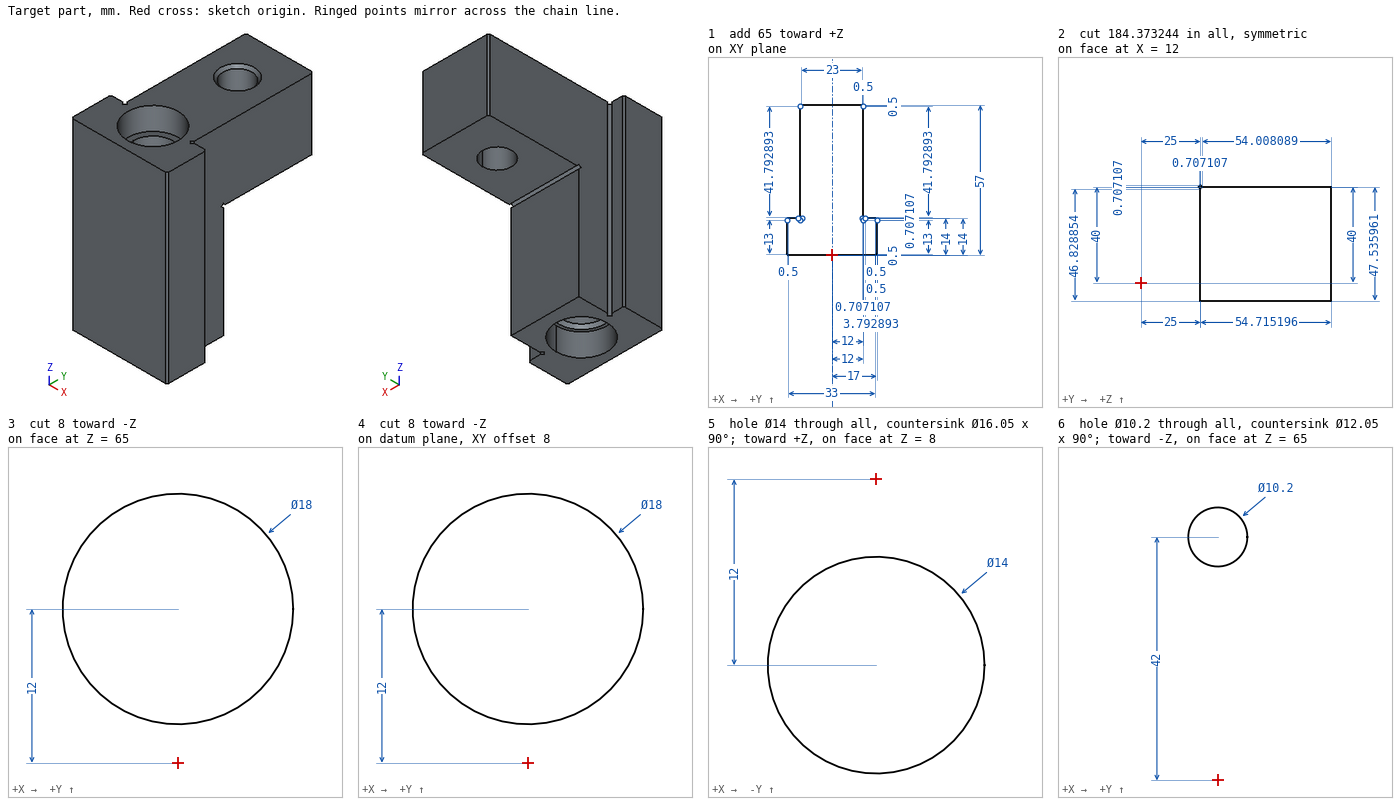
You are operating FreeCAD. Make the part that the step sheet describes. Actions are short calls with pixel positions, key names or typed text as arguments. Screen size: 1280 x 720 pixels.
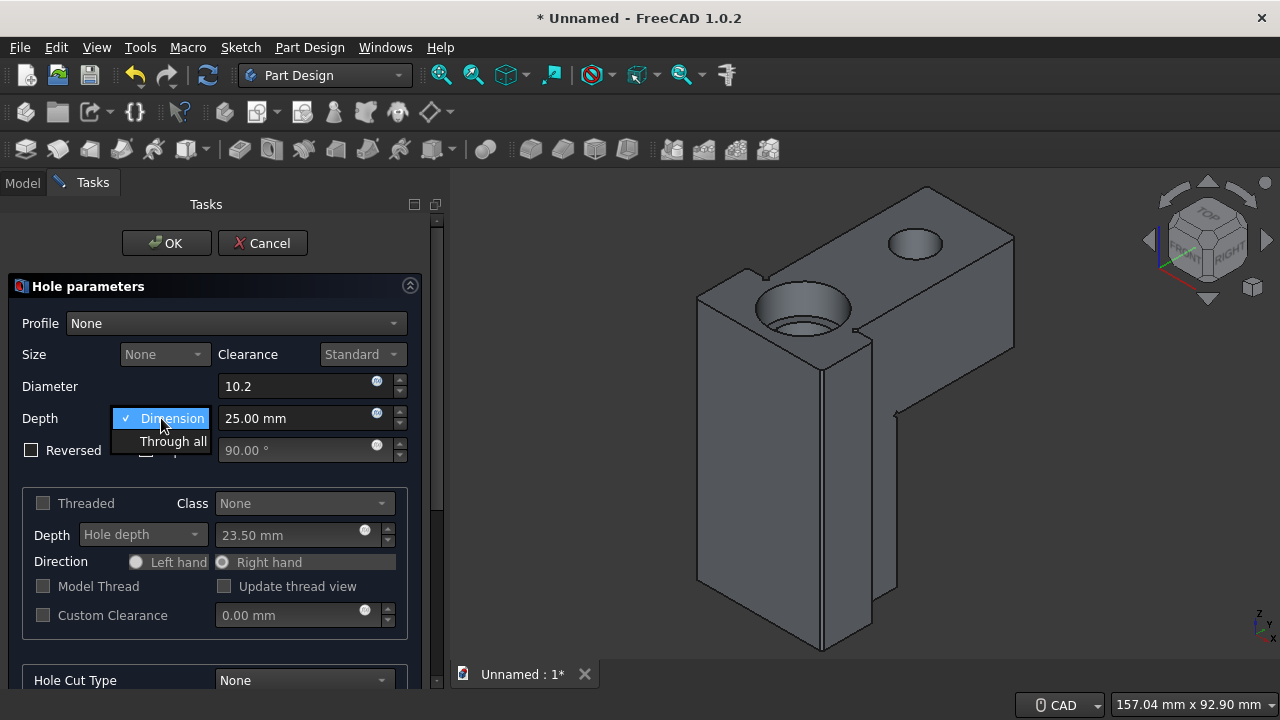
click(160, 442)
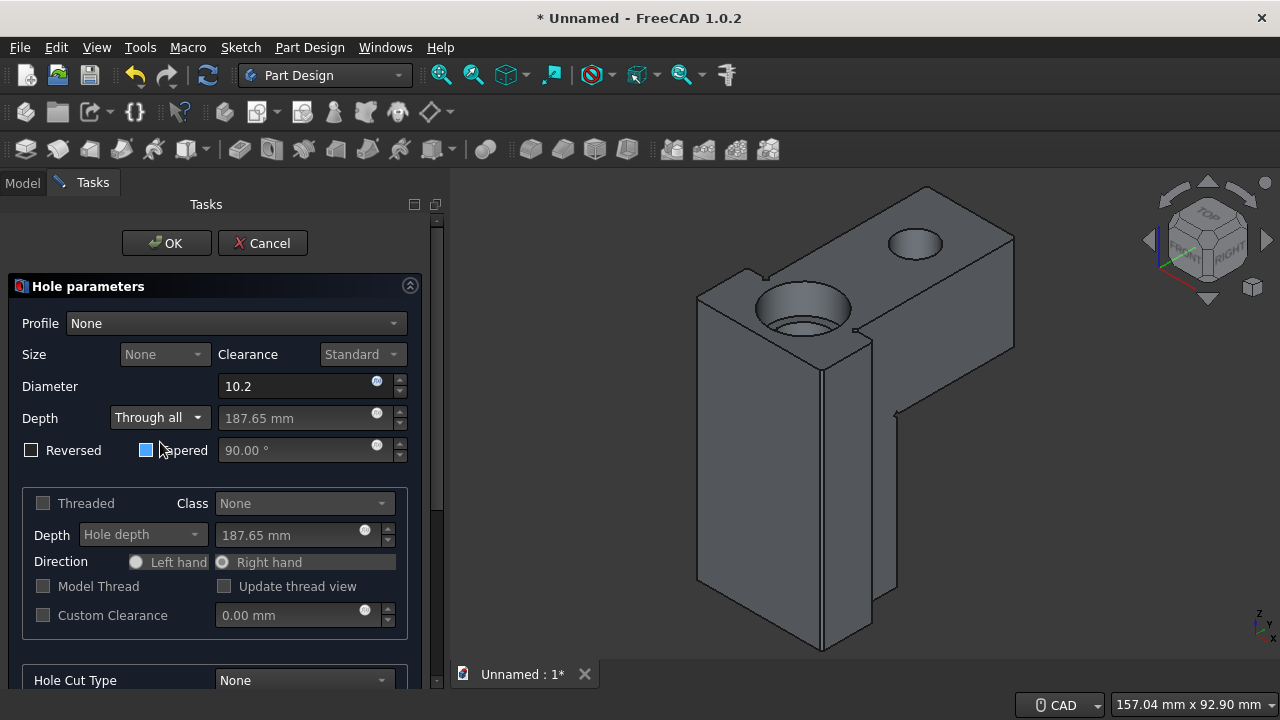
scroll(437, 451, down, 2)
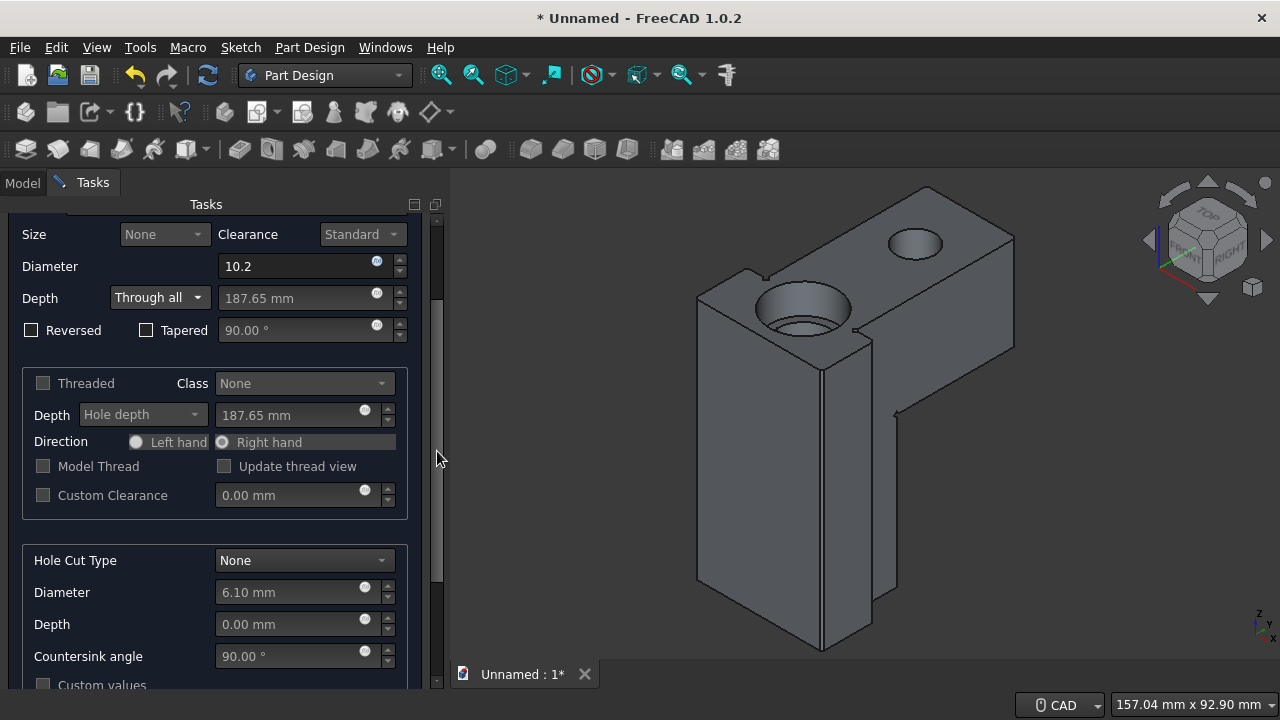
click(306, 560)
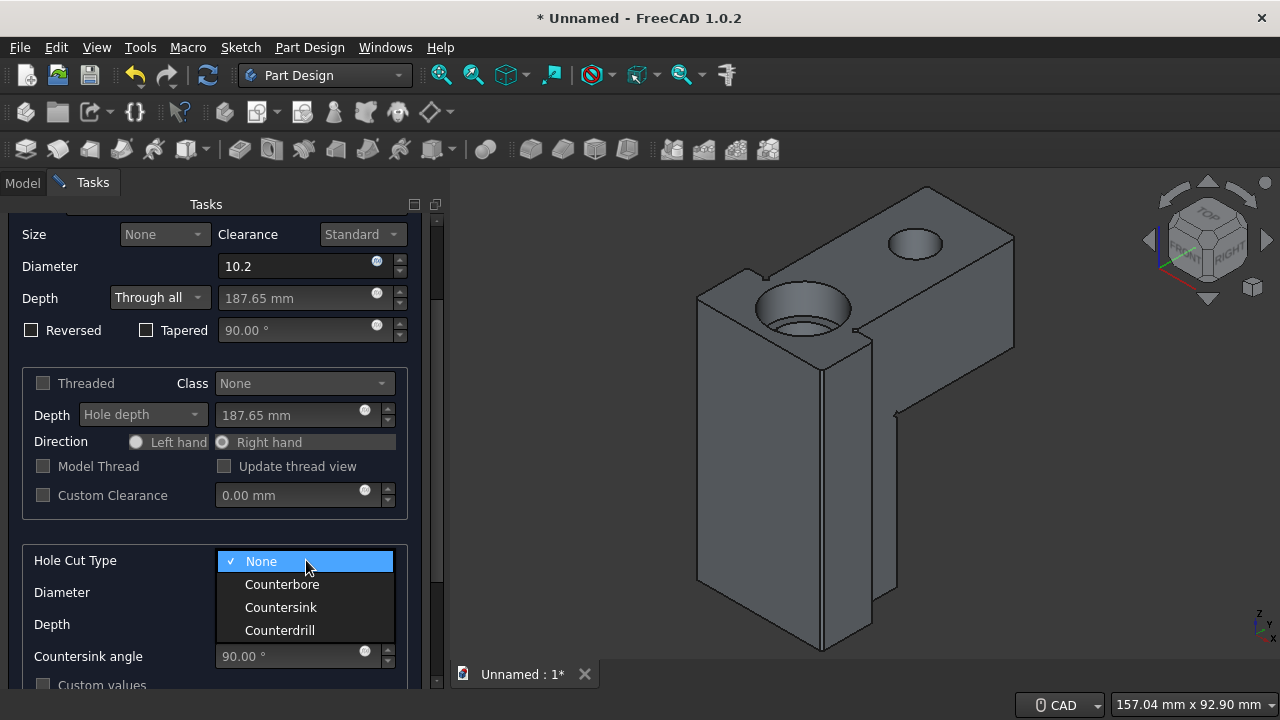
click(304, 608)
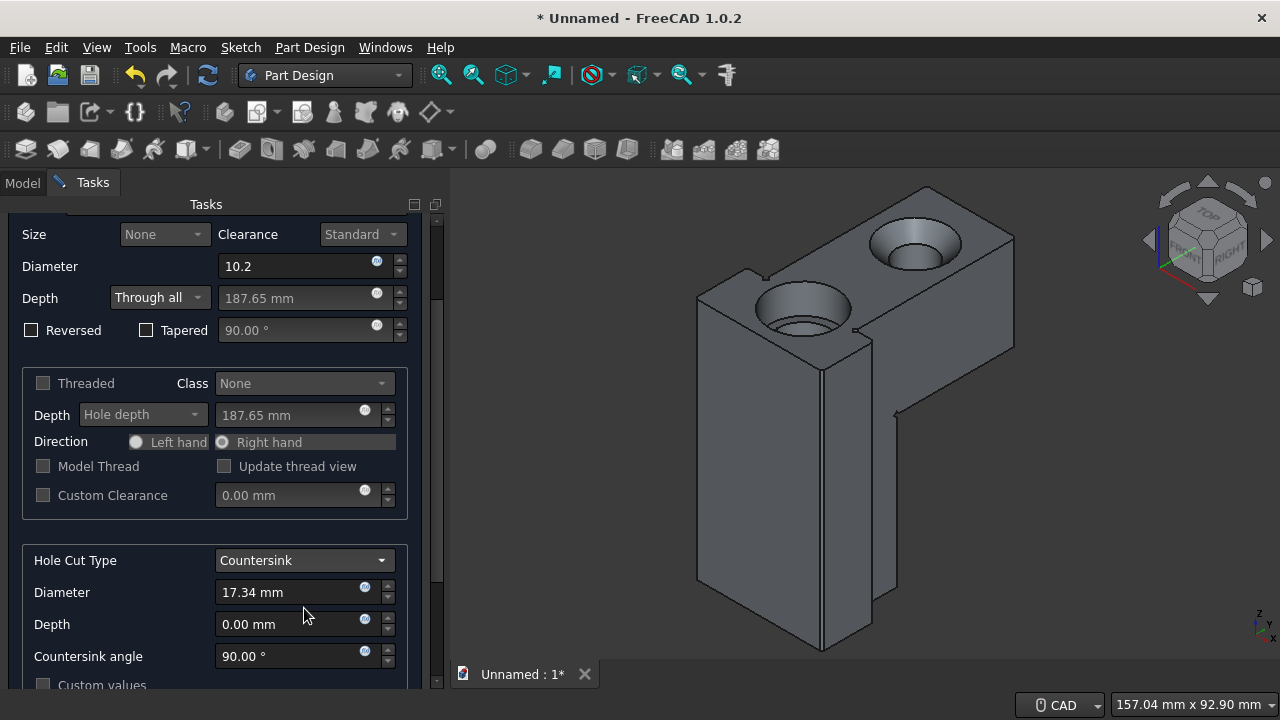
triple_click(298, 592)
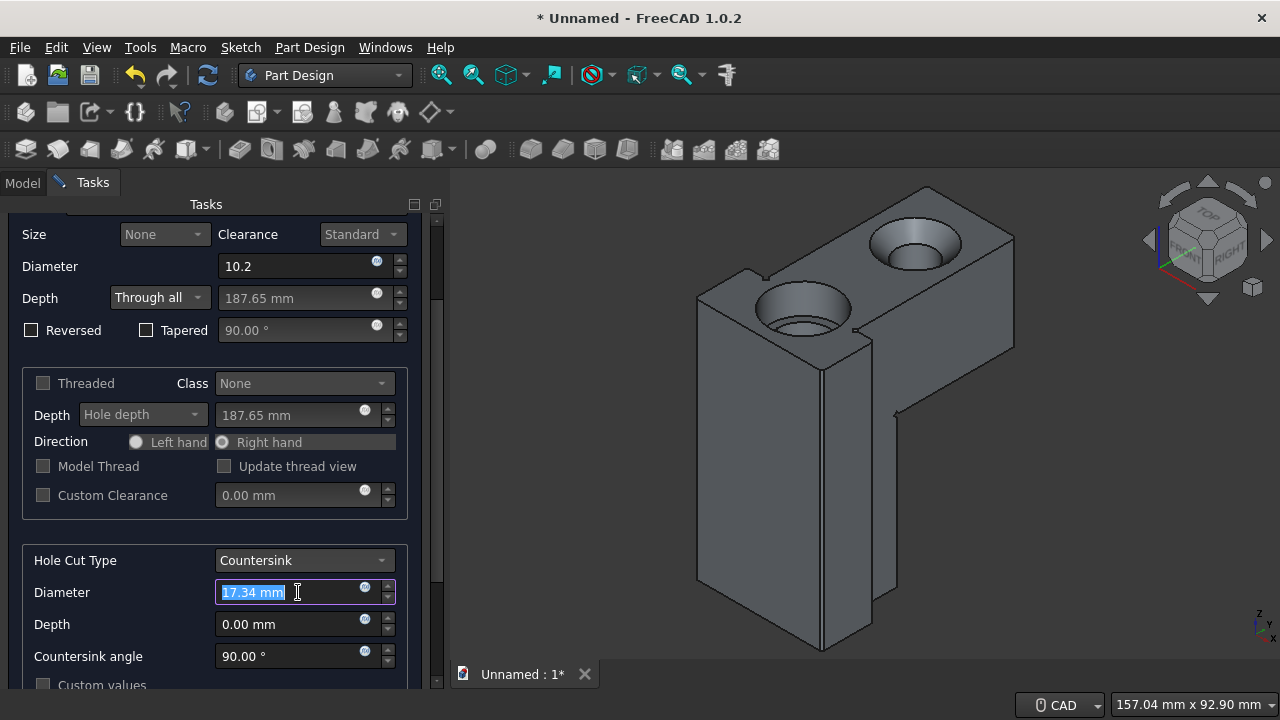
text(12.05)
key(Tab)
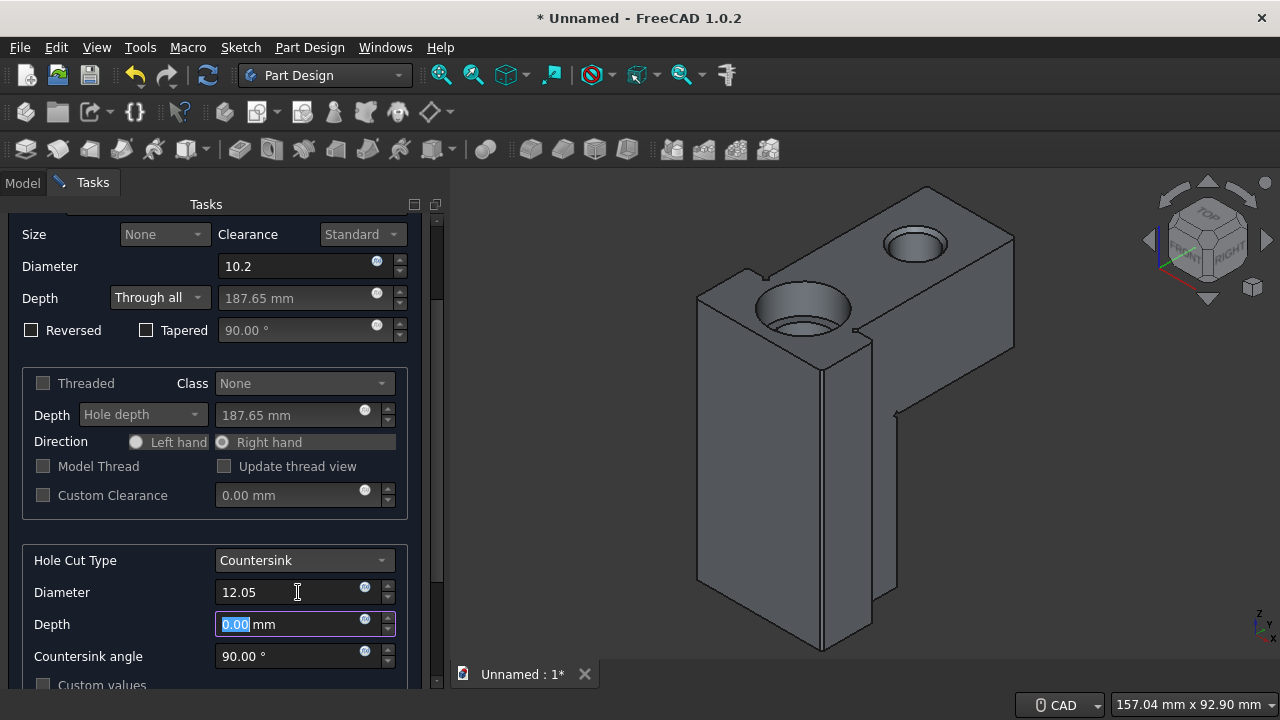
scroll(437, 451, up, 3)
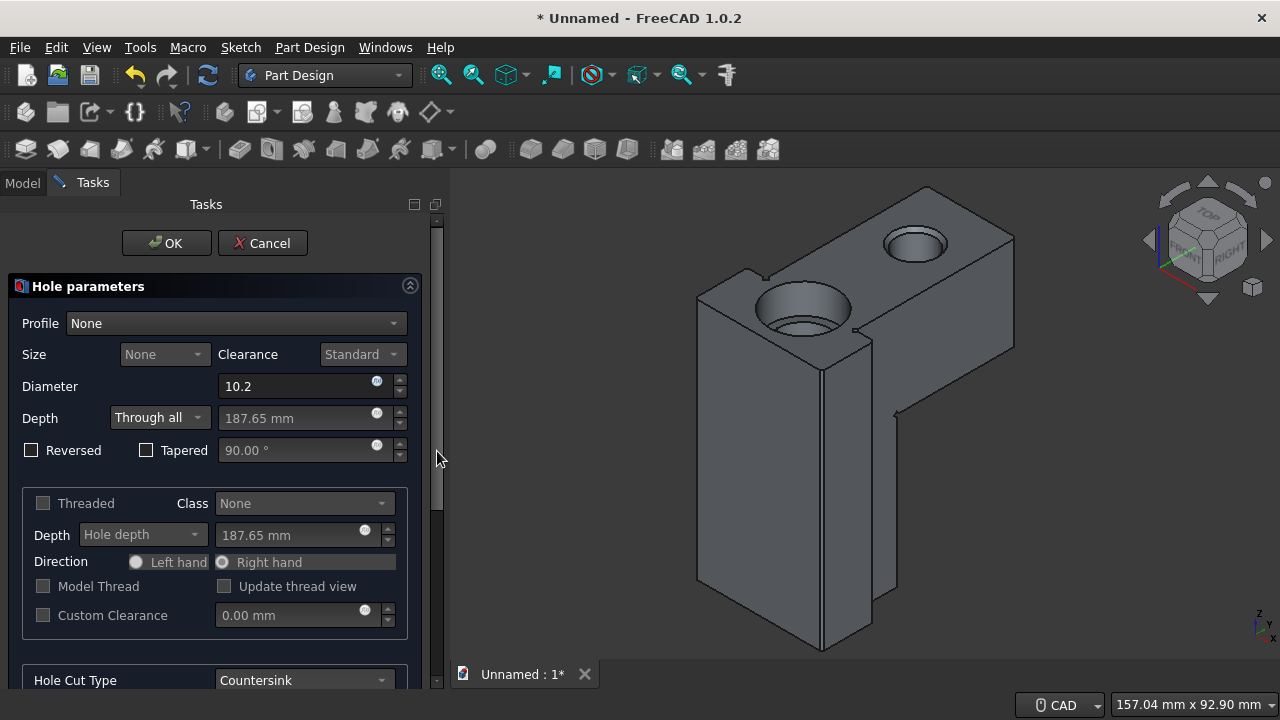
click(167, 243)